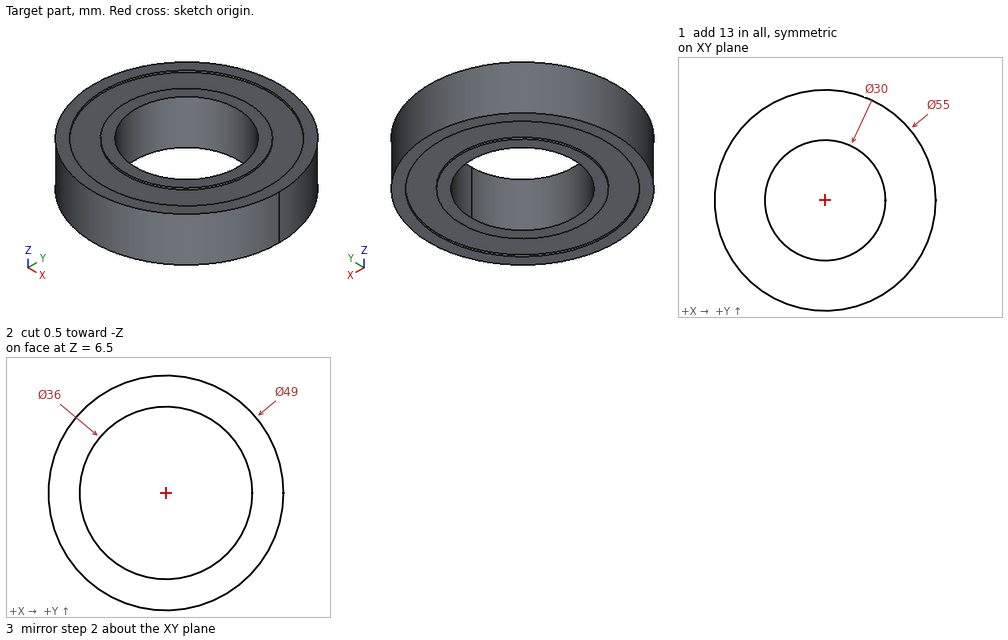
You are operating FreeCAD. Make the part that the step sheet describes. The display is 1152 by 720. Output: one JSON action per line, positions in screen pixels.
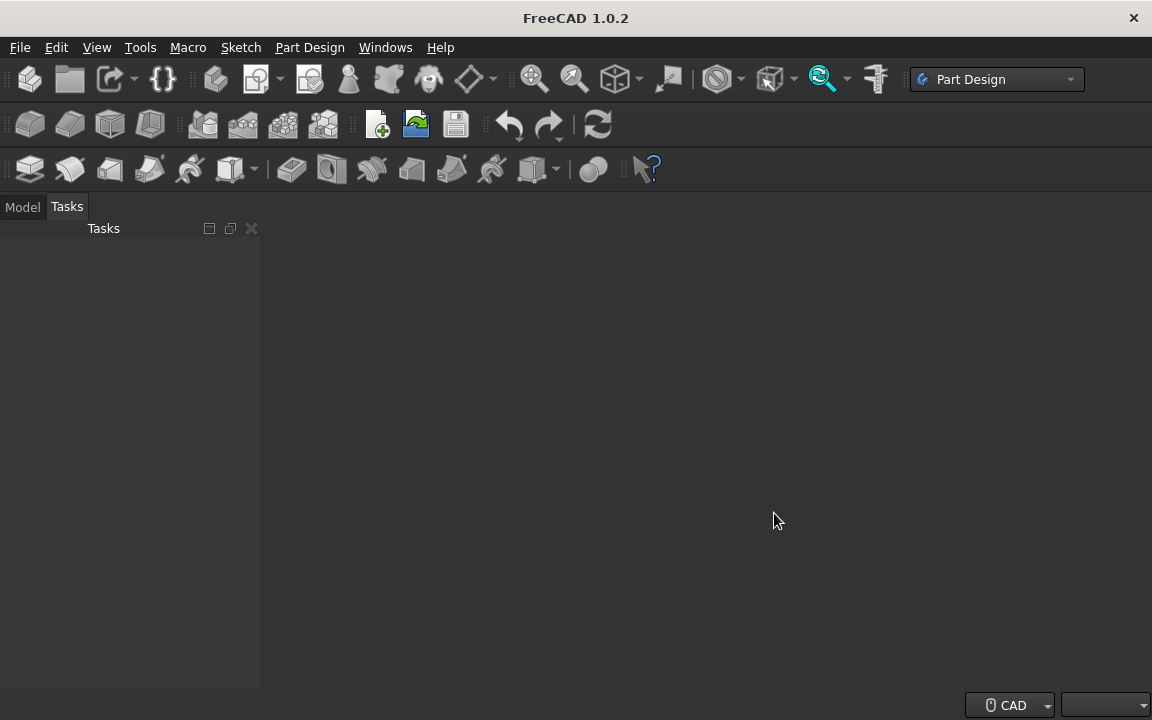
{"action": "left_click", "coordinate": [376, 124]}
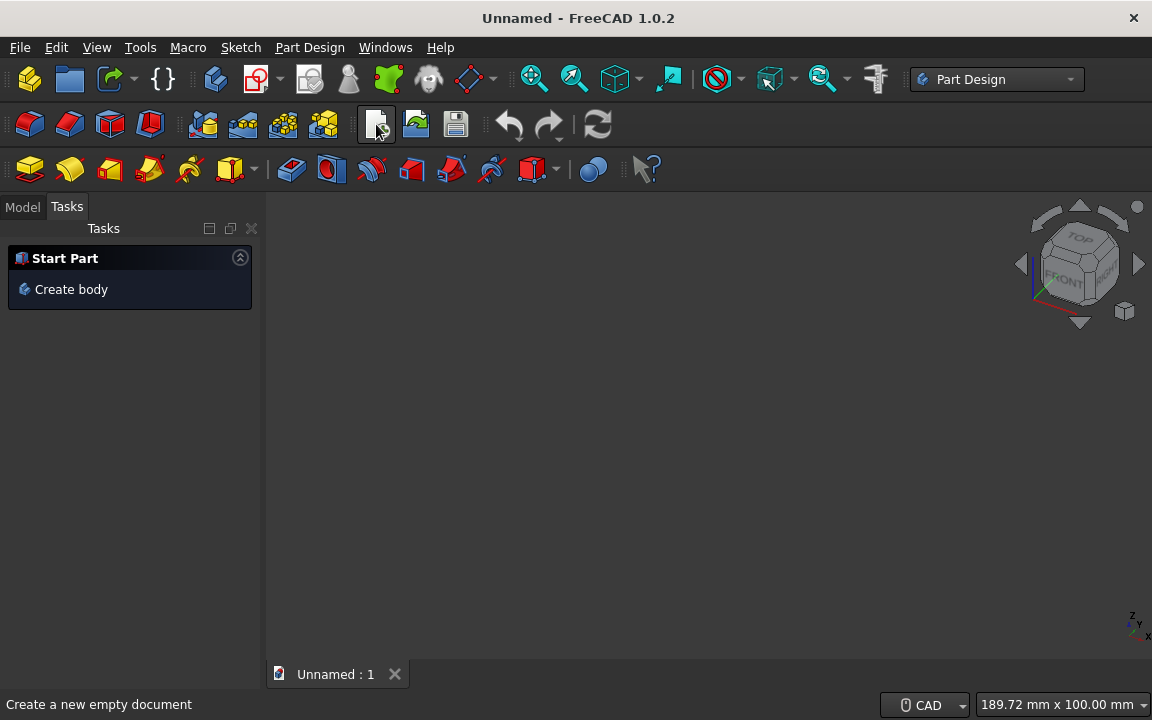
{"action": "left_click", "coordinate": [256, 80]}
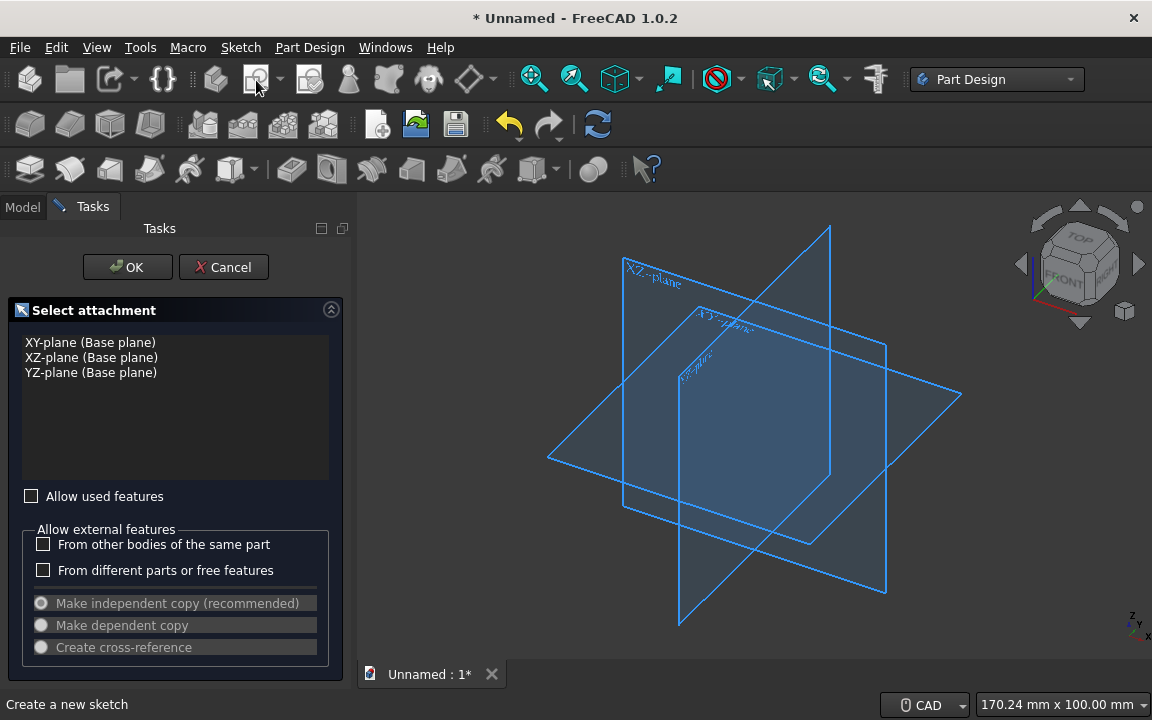
{"action": "left_click", "coordinate": [82, 342]}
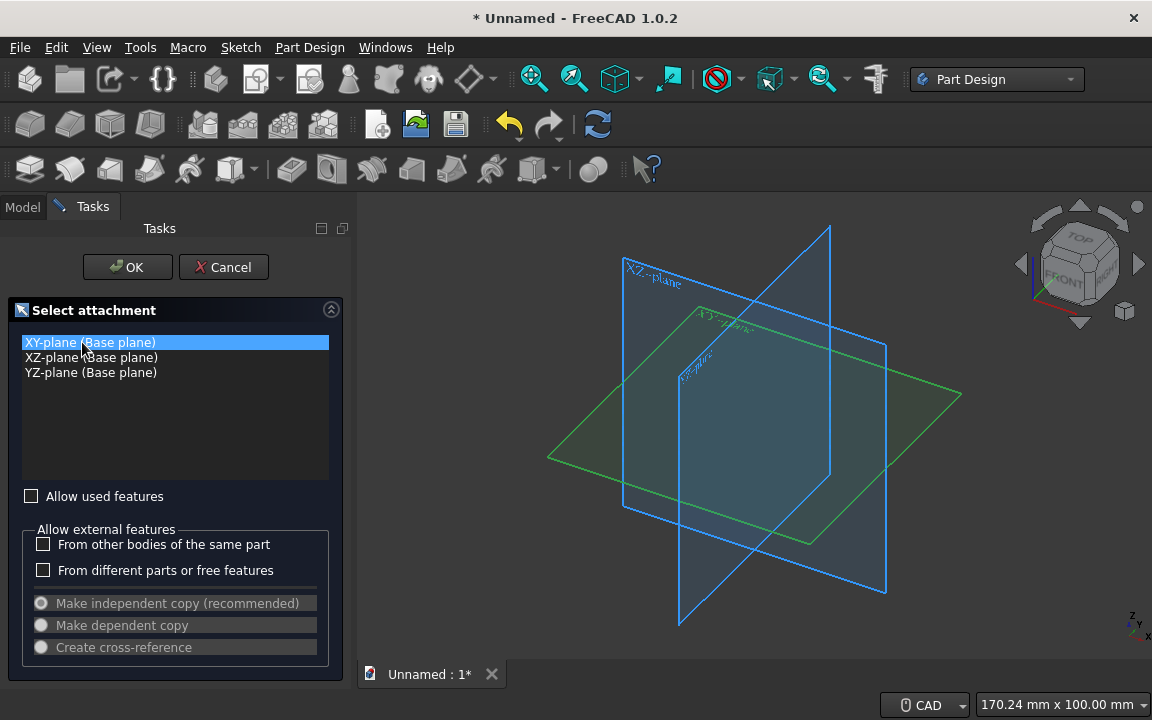
{"action": "left_click", "coordinate": [128, 267]}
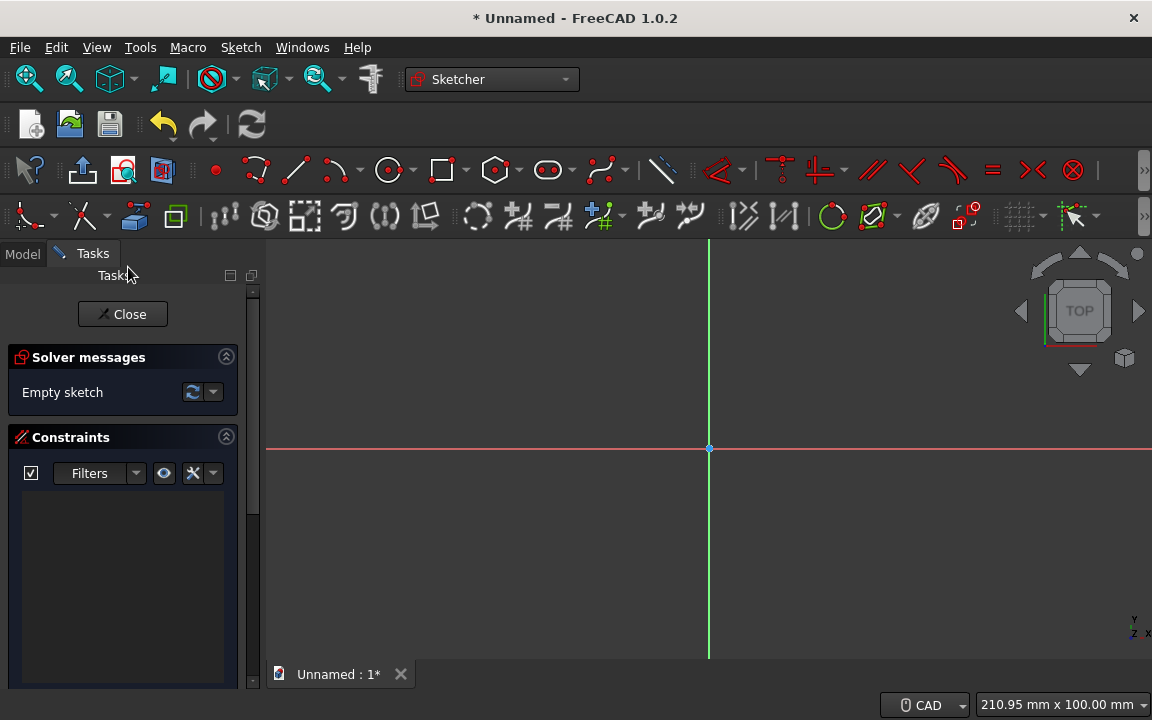
{"action": "key", "text": "g c"}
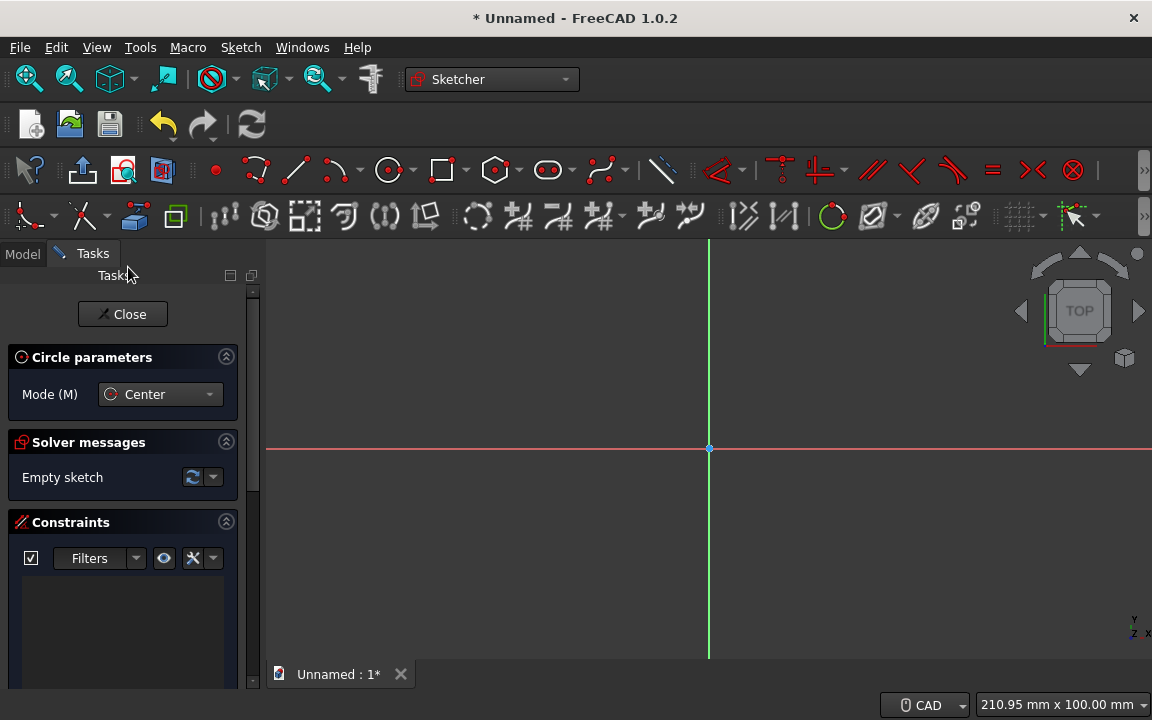
{"action": "left_click", "coordinate": [709, 449]}
{"action": "left_click", "coordinate": [791, 367]}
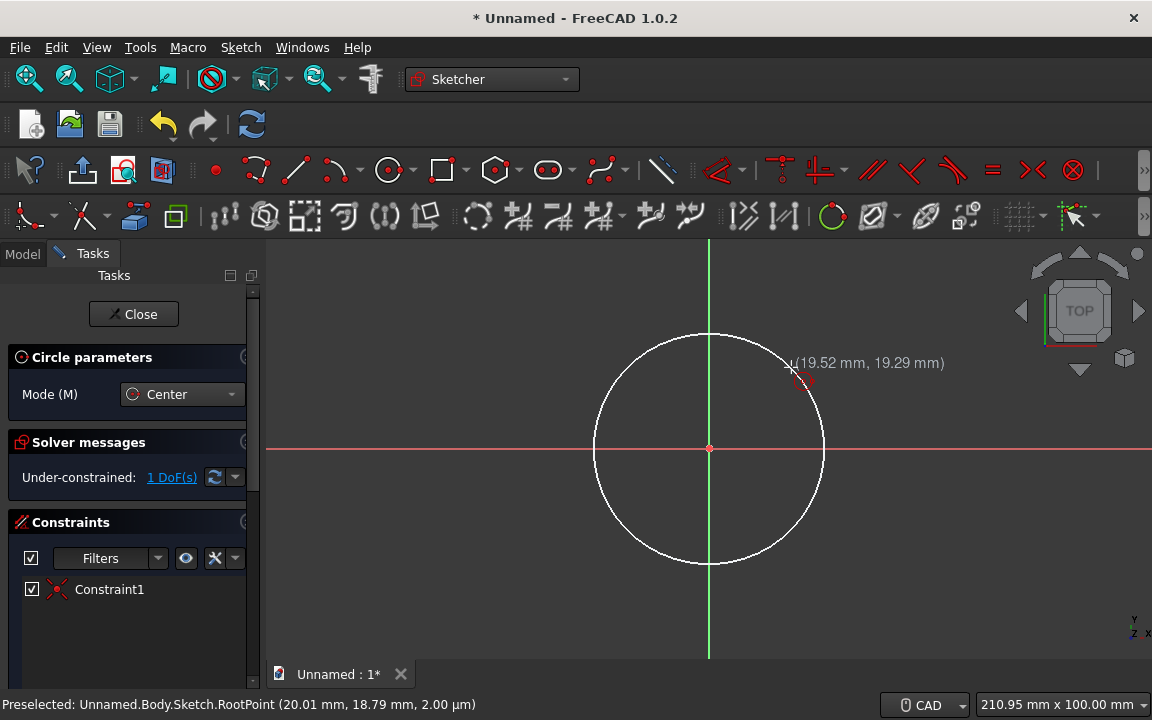
{"action": "left_click", "coordinate": [709, 449]}
{"action": "left_click", "coordinate": [754, 404]}
{"action": "key", "text": "Escape"}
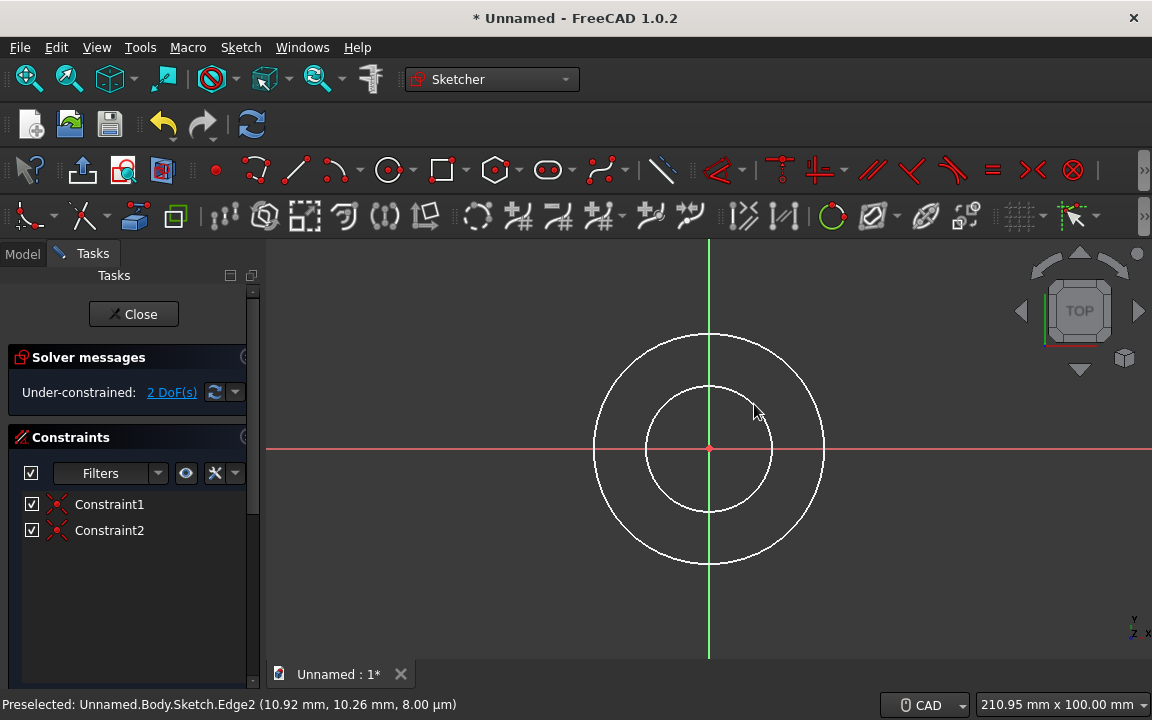
{"action": "left_click", "coordinate": [718, 170]}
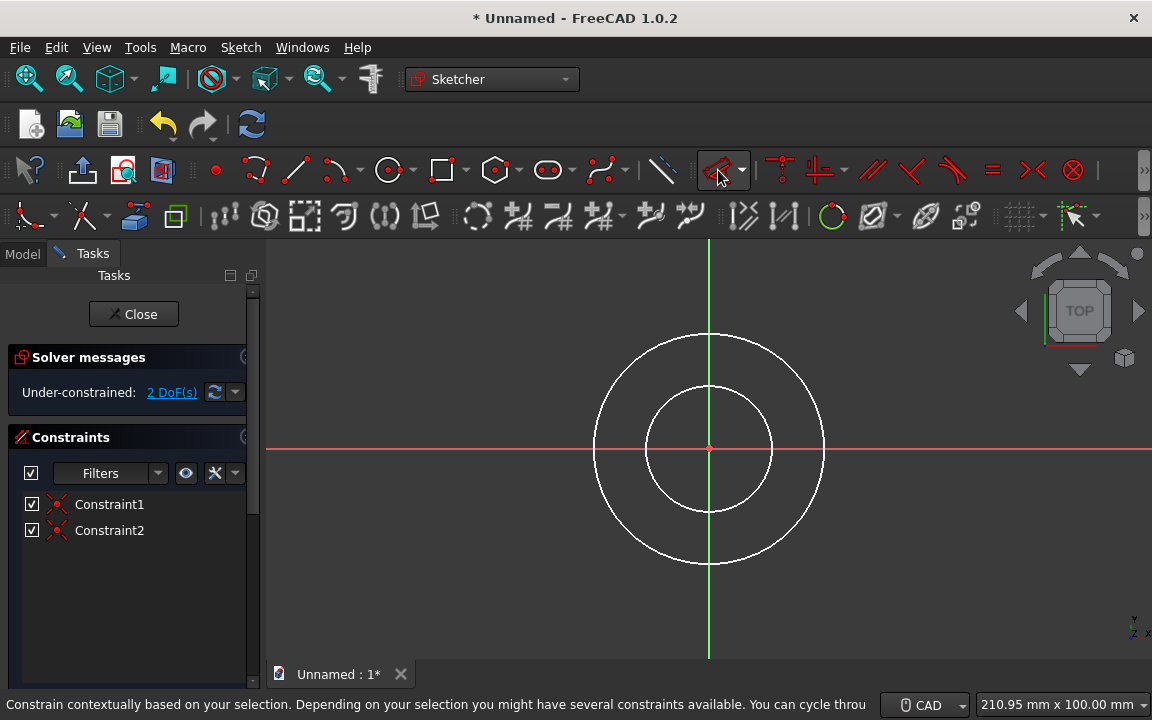
{"action": "left_click", "coordinate": [790, 367]}
{"action": "left_click", "coordinate": [812, 344]}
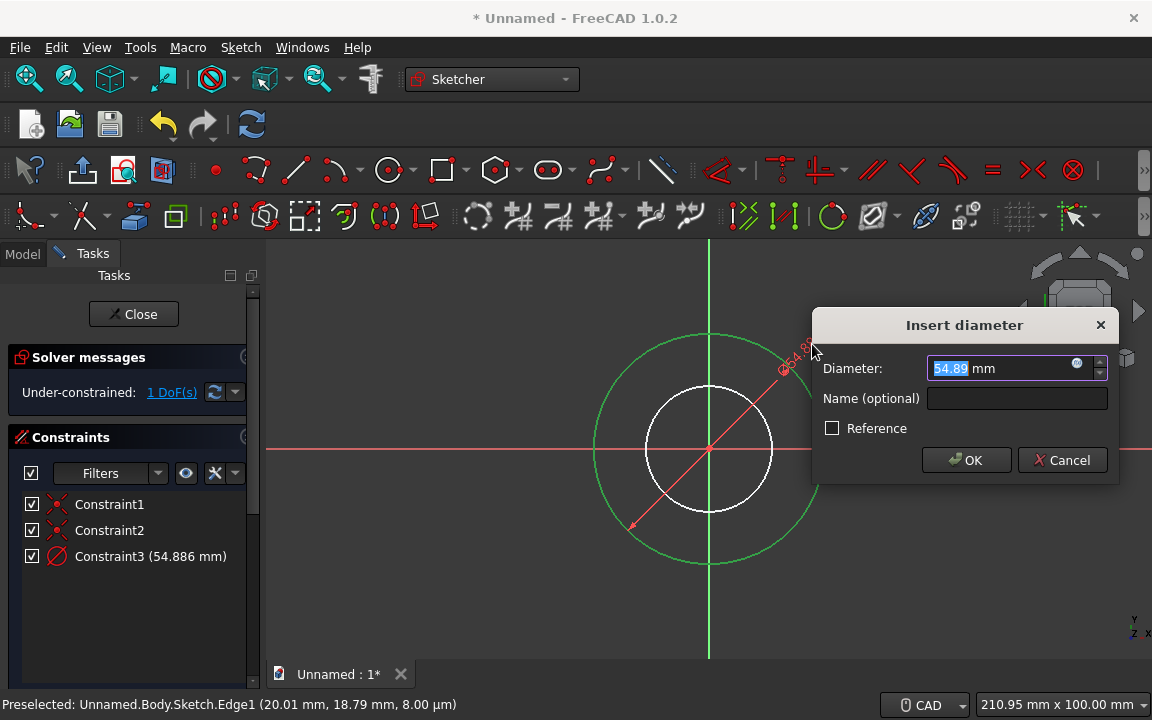
{"action": "type", "text": "55"}
{"action": "key", "text": "Return"}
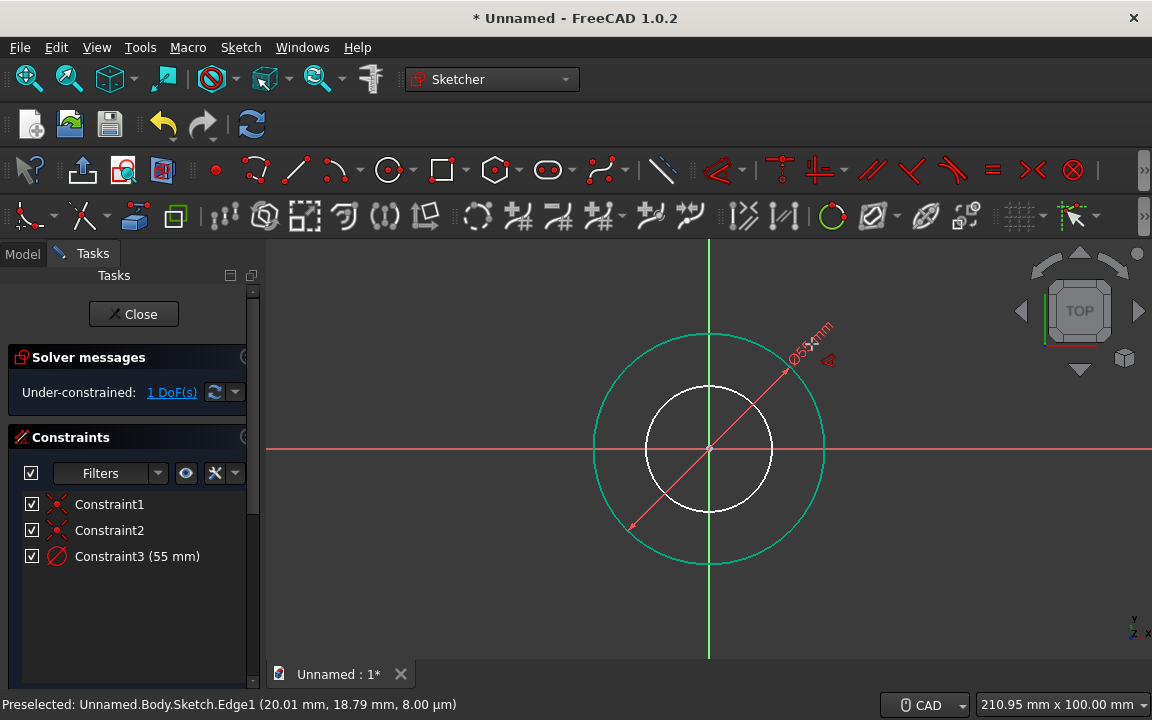
{"action": "left_click", "coordinate": [753, 404]}
{"action": "left_click", "coordinate": [775, 381]}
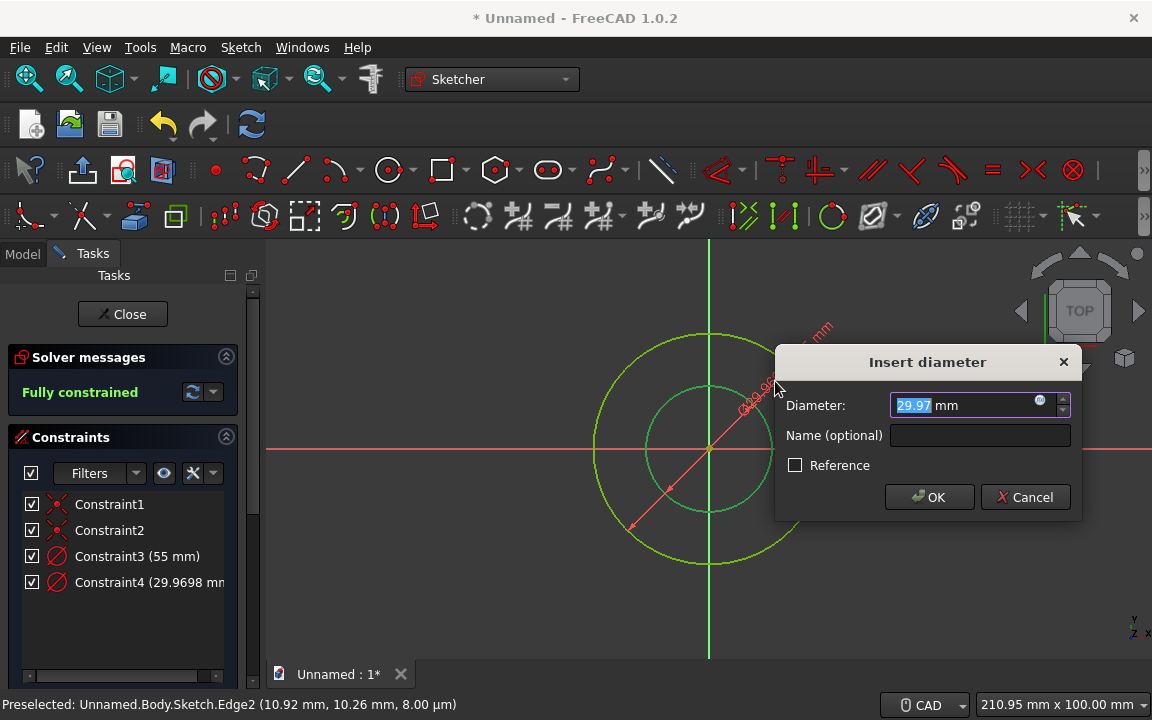
{"action": "type", "text": "30"}
{"action": "key", "text": "Return"}
{"action": "key", "text": "Escape"}